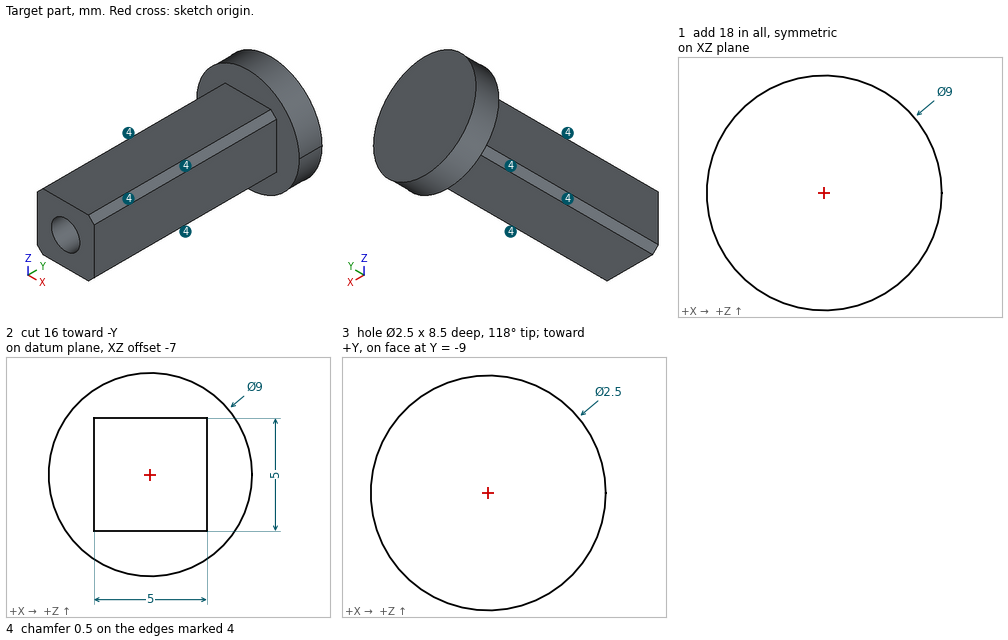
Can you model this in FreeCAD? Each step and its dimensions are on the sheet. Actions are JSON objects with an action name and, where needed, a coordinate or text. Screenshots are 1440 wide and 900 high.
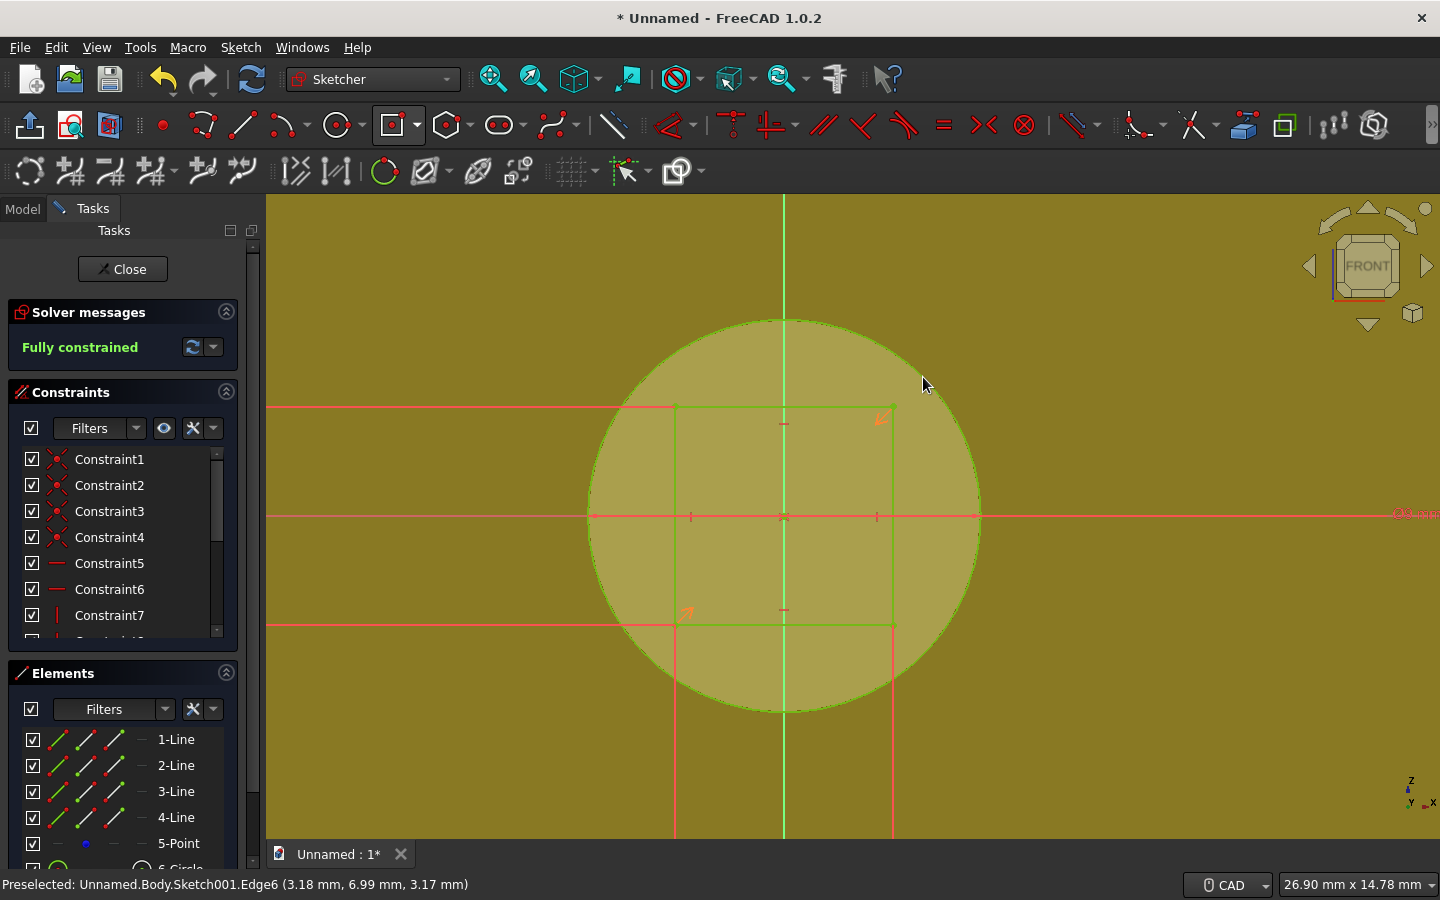
{"action": "left_click", "coordinate": [123, 269]}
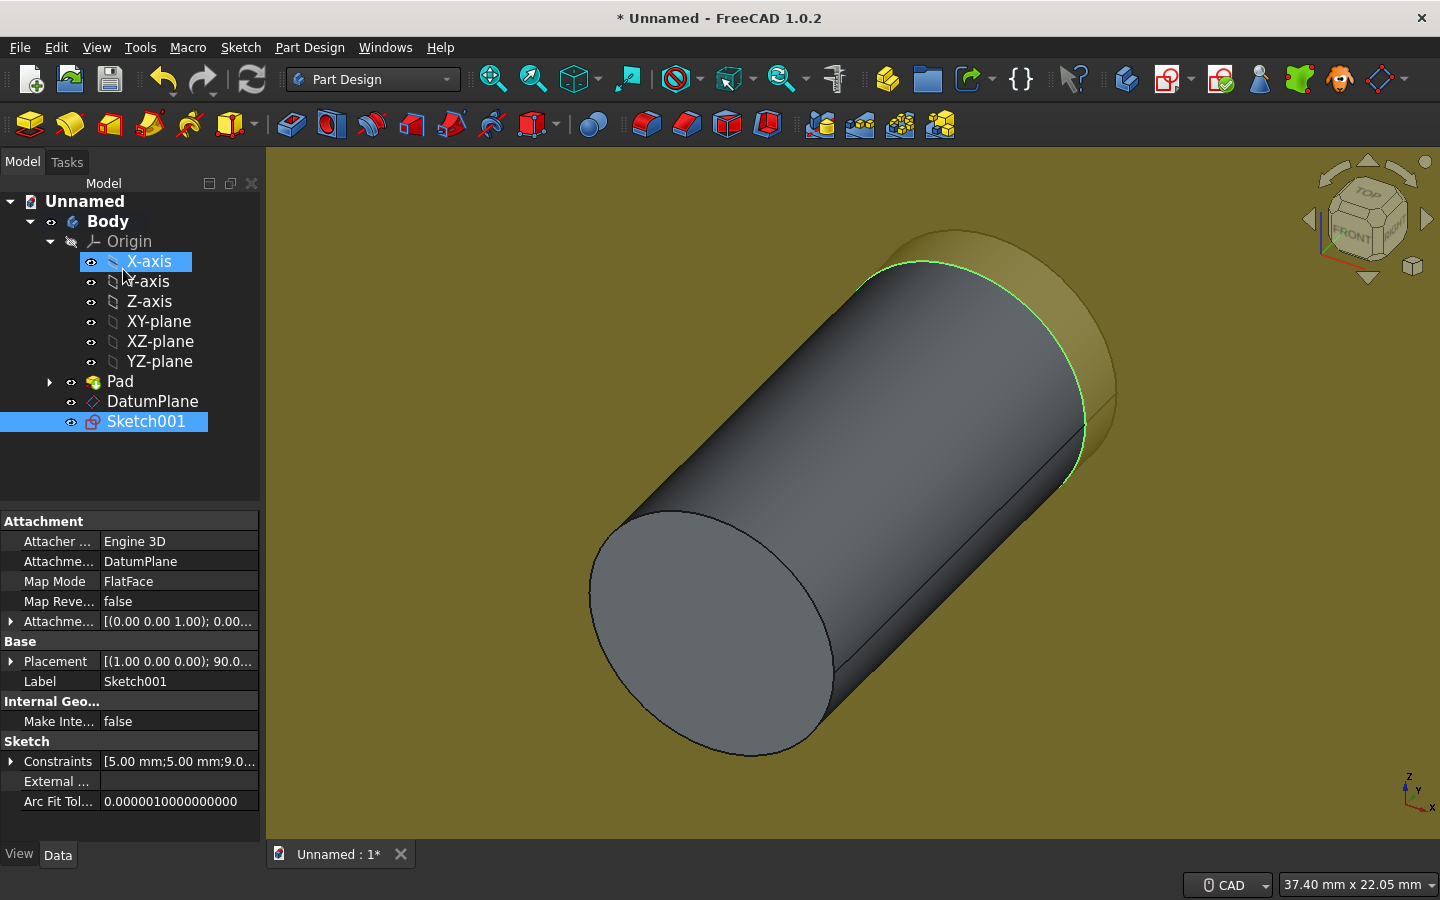
{"action": "left_click", "coordinate": [292, 124]}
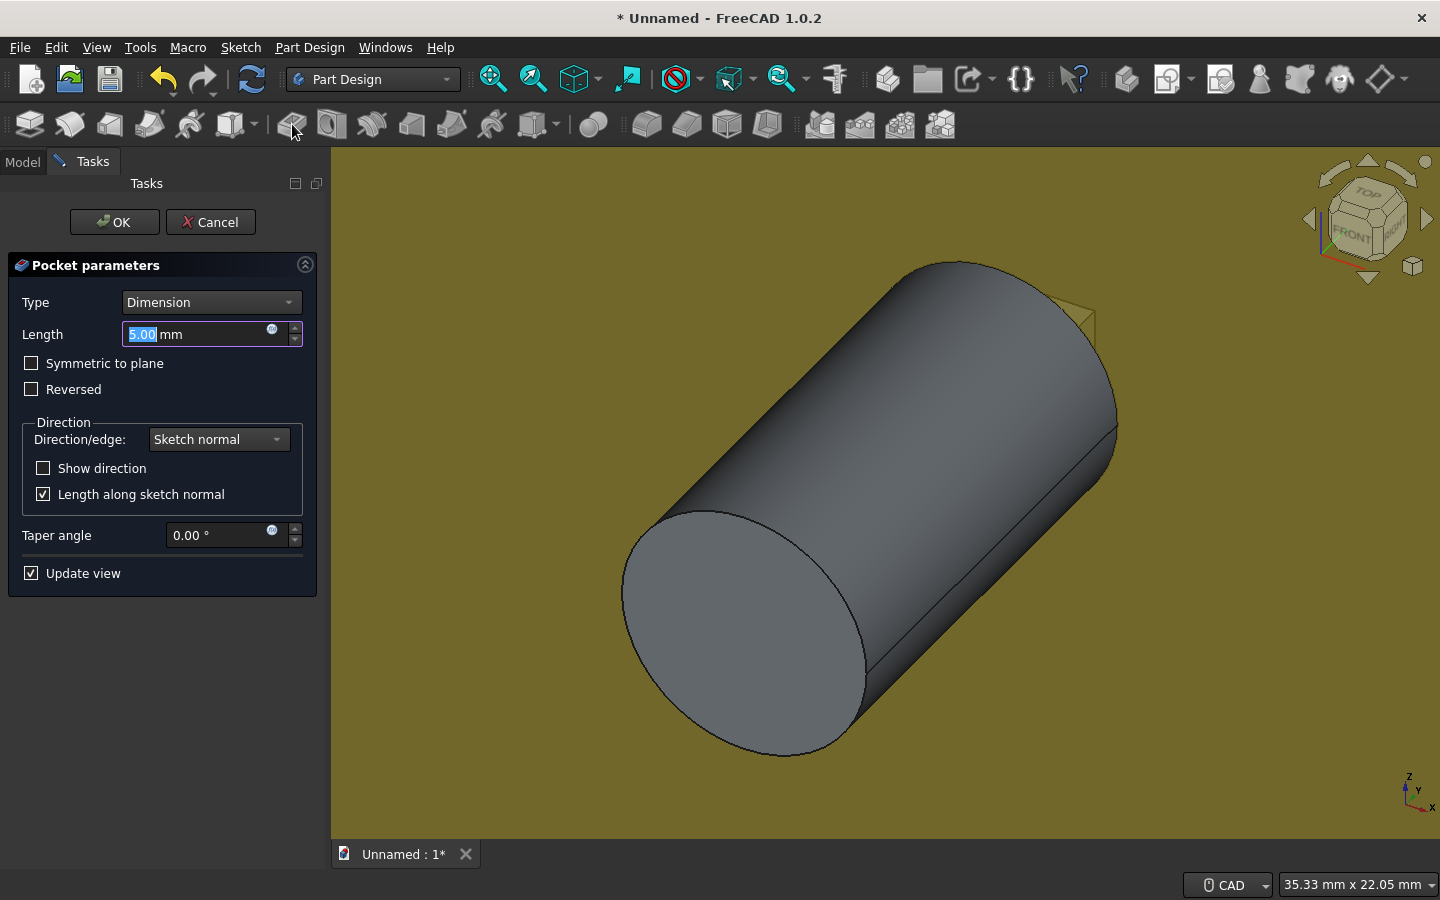
{"action": "type", "text": "16"}
{"action": "key", "text": "Tab"}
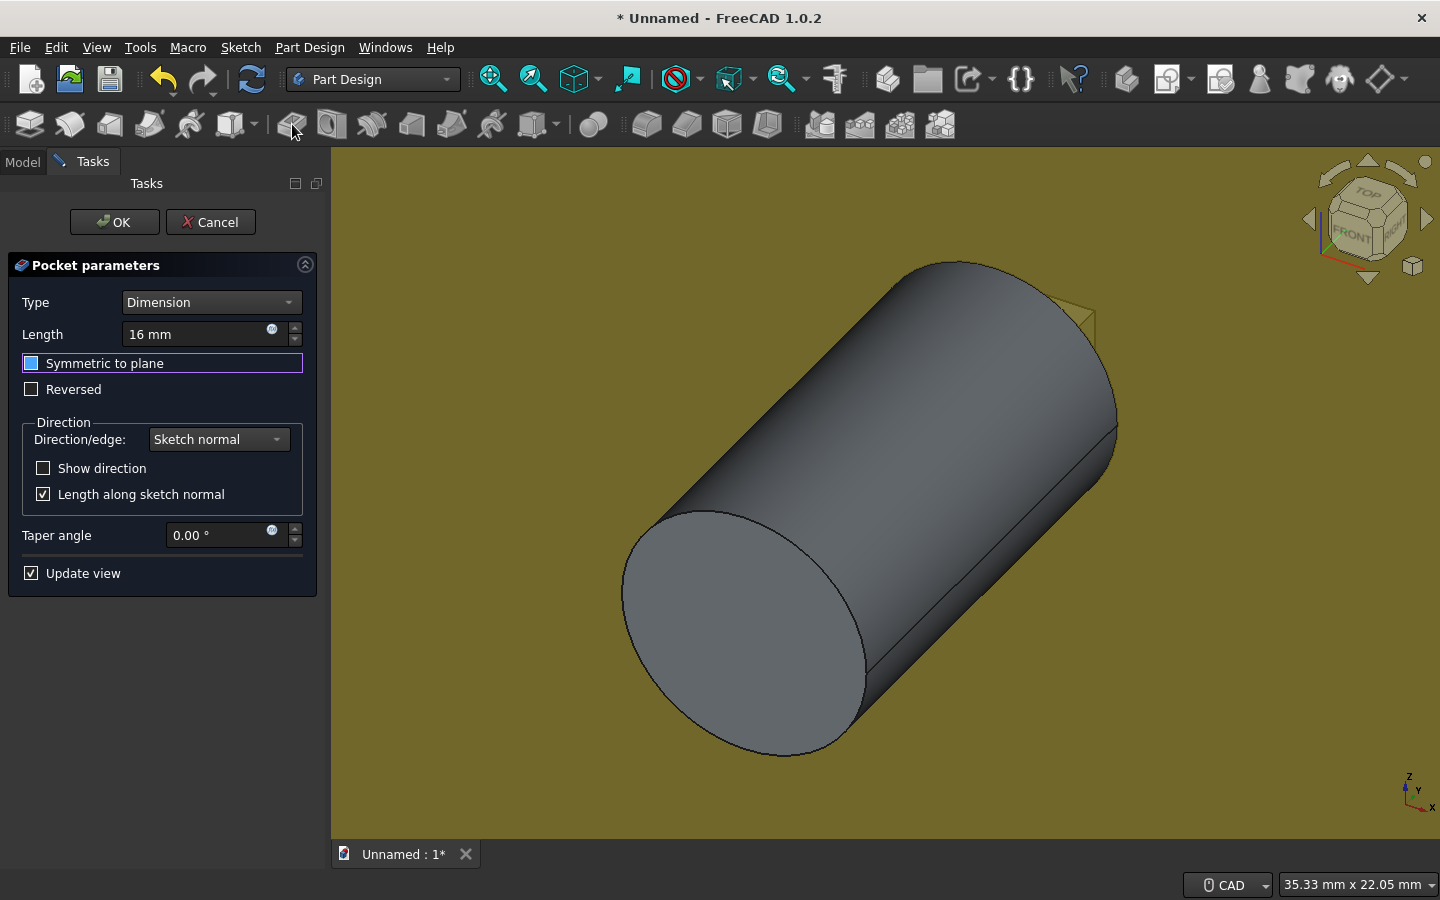
{"action": "left_click", "coordinate": [30, 389]}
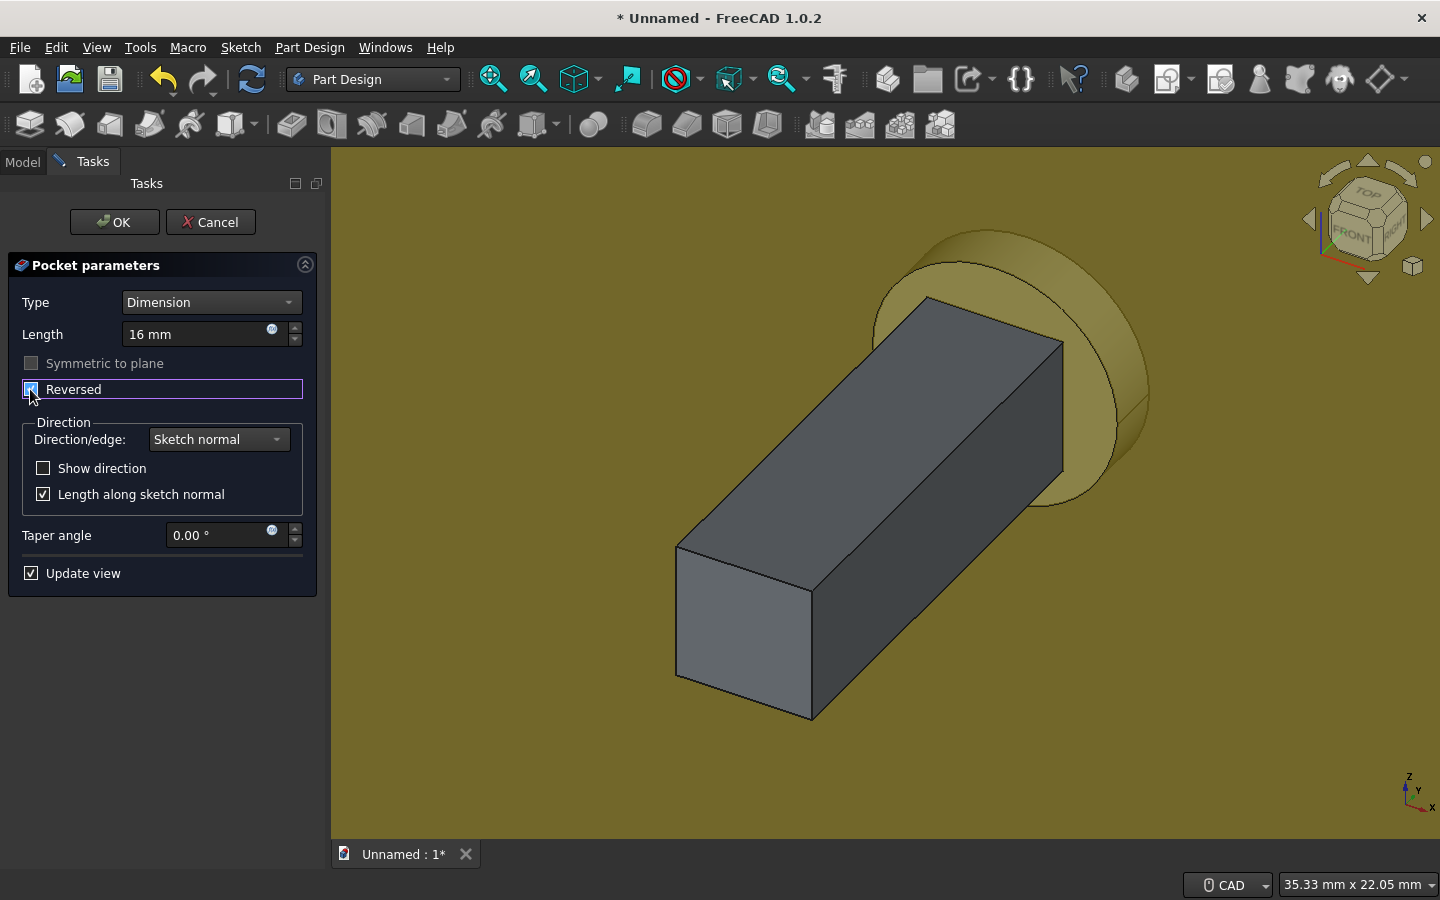
{"action": "left_click", "coordinate": [115, 222]}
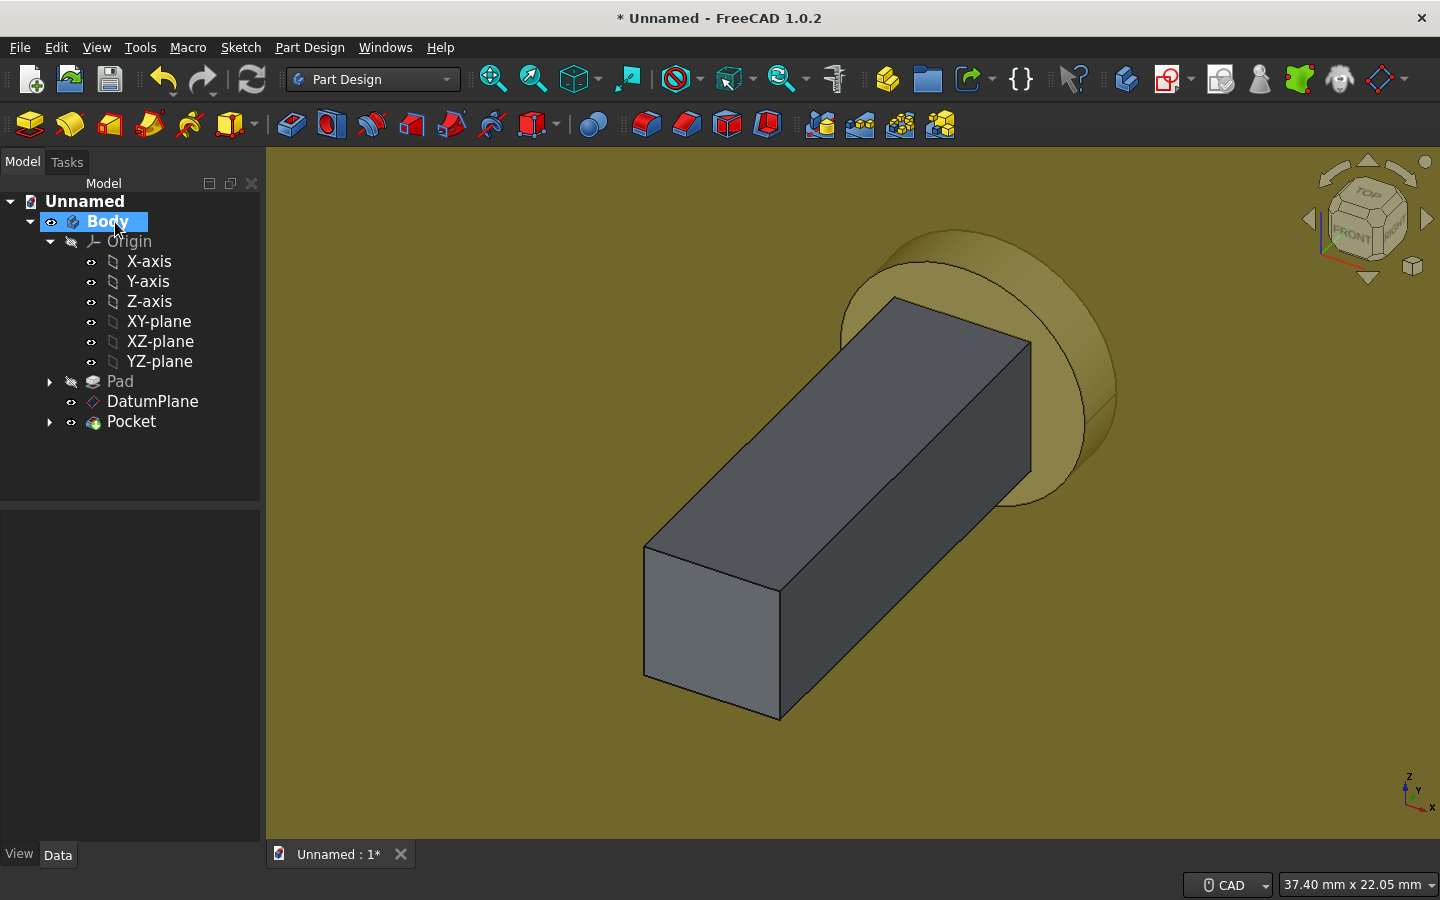
{"action": "left_click", "coordinate": [116, 402]}
{"action": "key", "text": "space"}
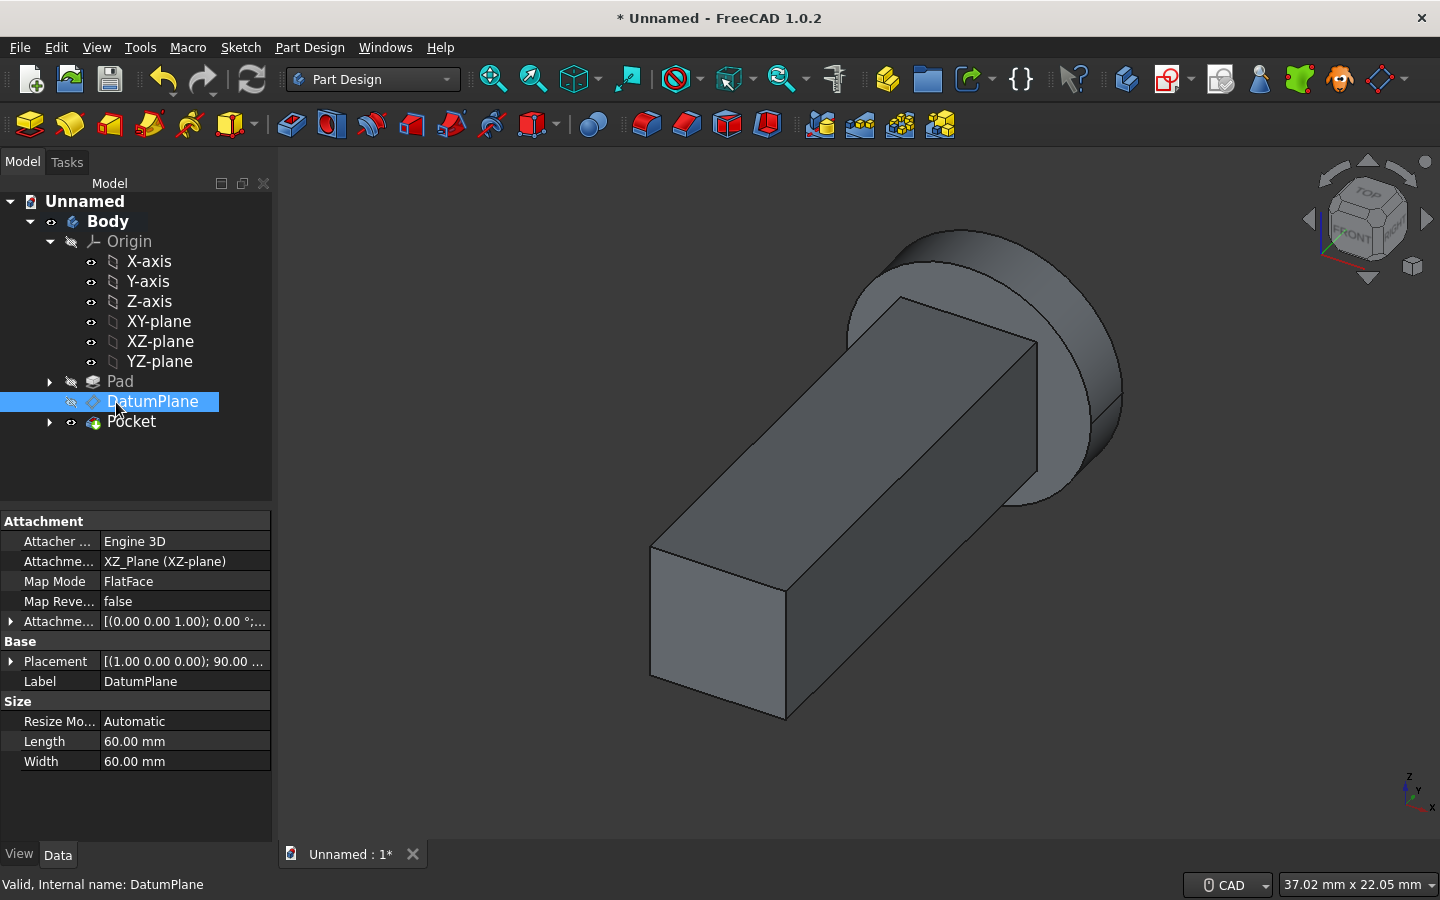
{"action": "left_click", "coordinate": [718, 632]}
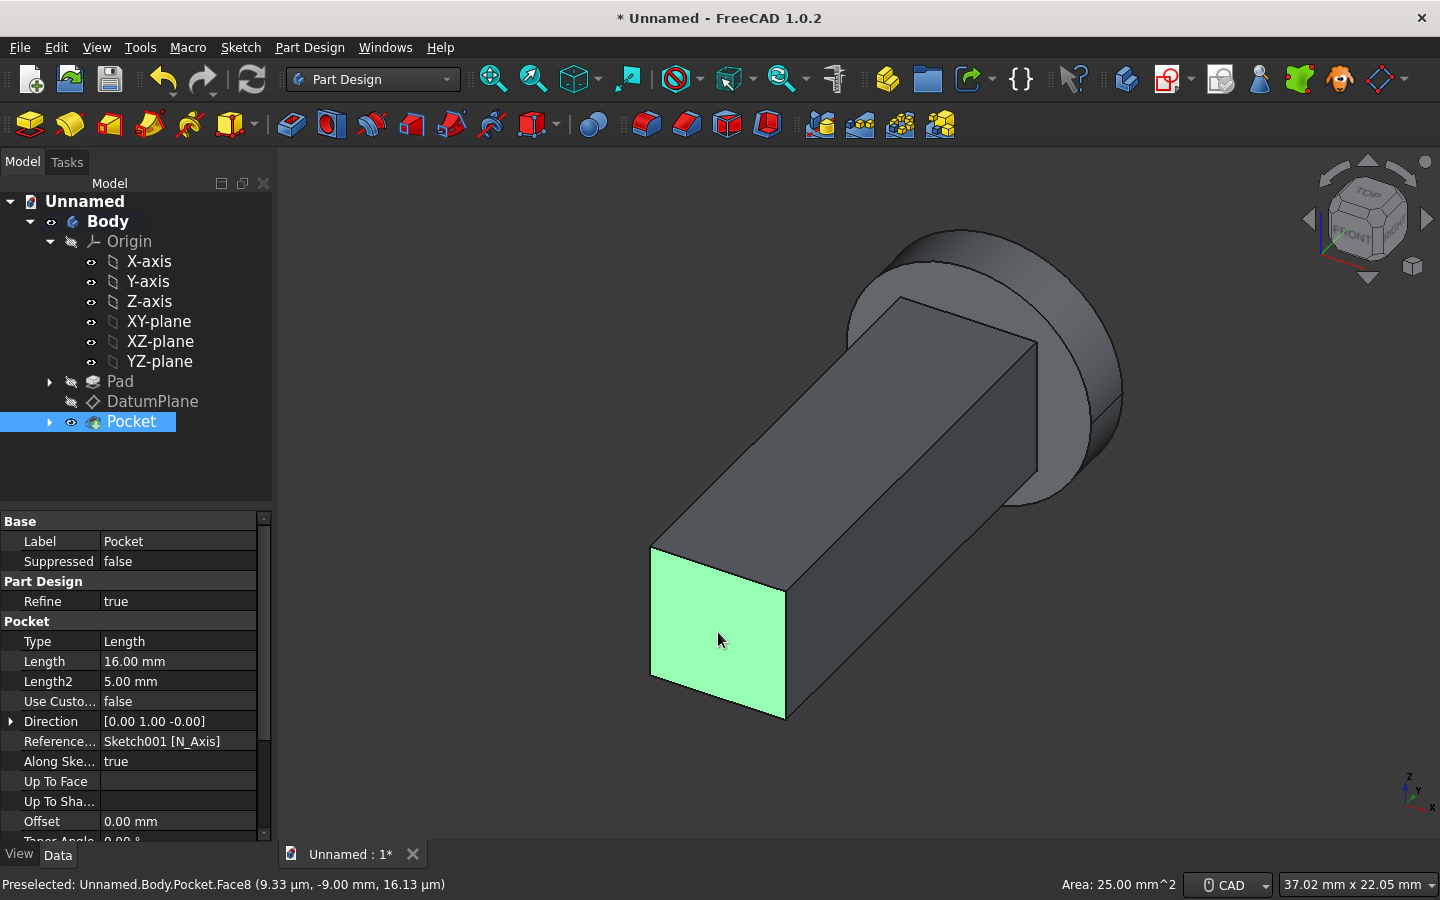
{"action": "left_click", "coordinate": [1168, 80]}